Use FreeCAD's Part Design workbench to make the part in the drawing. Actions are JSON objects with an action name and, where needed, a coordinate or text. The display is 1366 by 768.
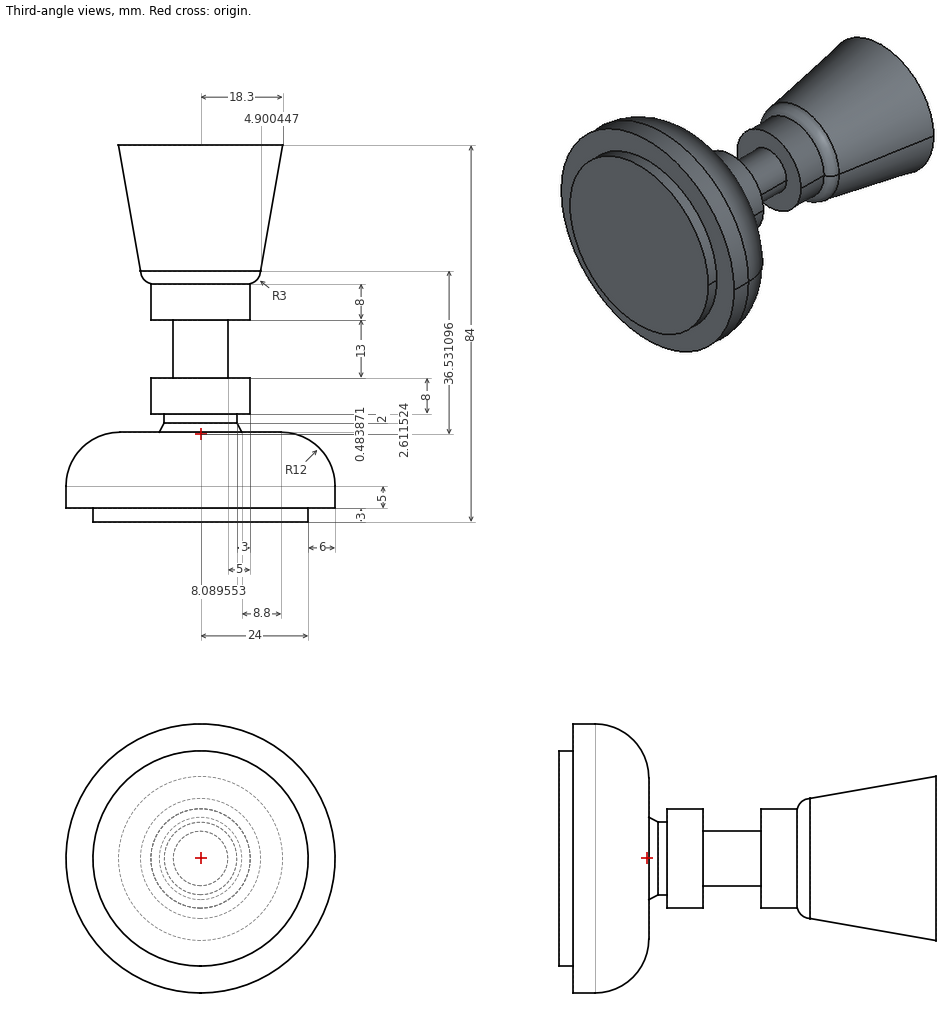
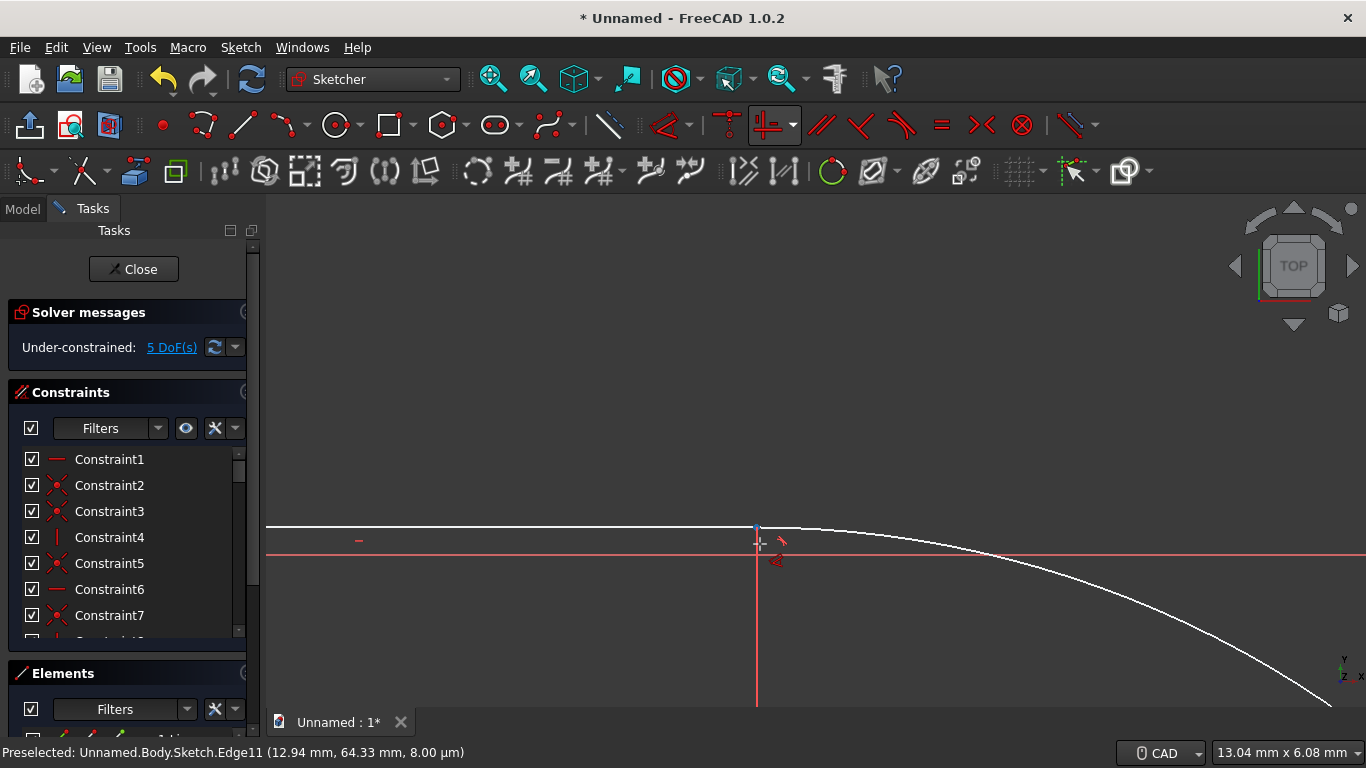
{"action": "left_click", "coordinate": [757, 527]}
{"action": "left_click", "coordinate": [791, 541]}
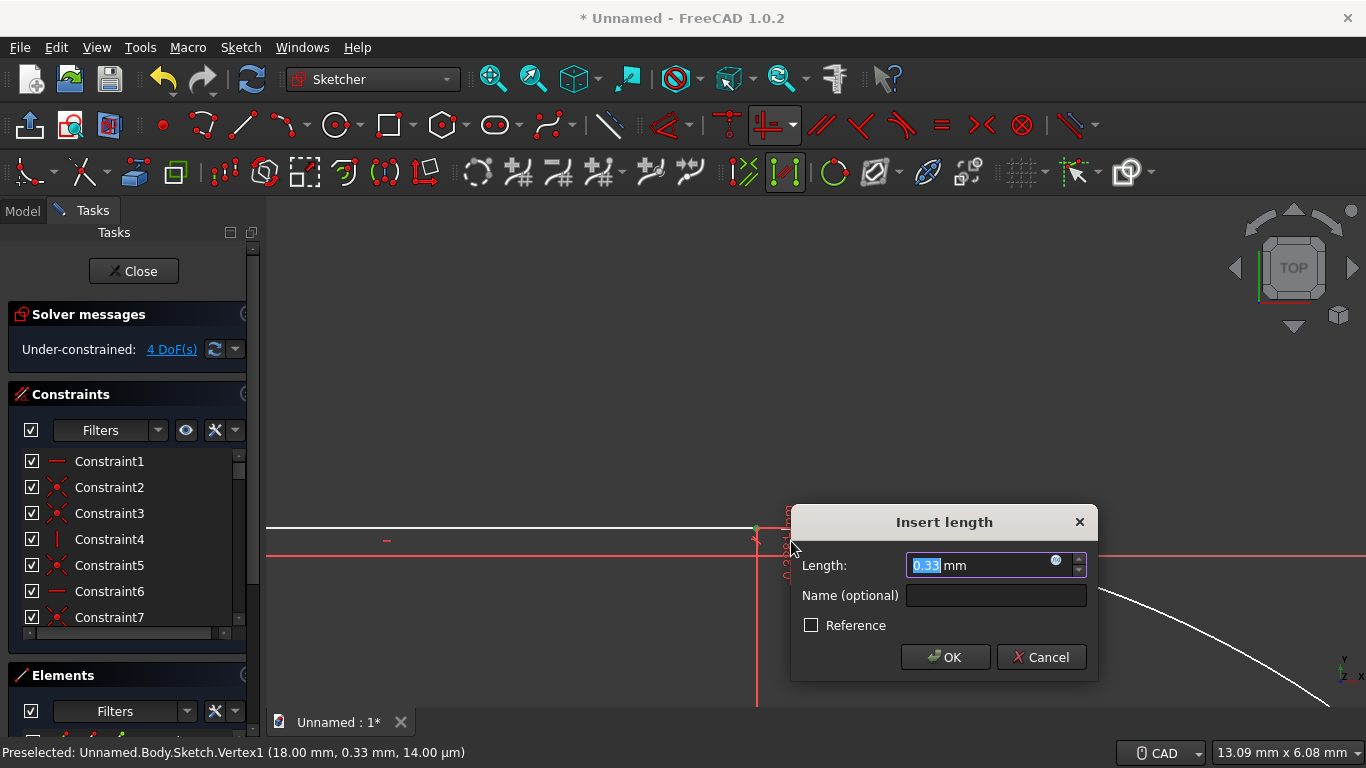
{"action": "type", "text": "0.483871"}
{"action": "key", "text": "Return"}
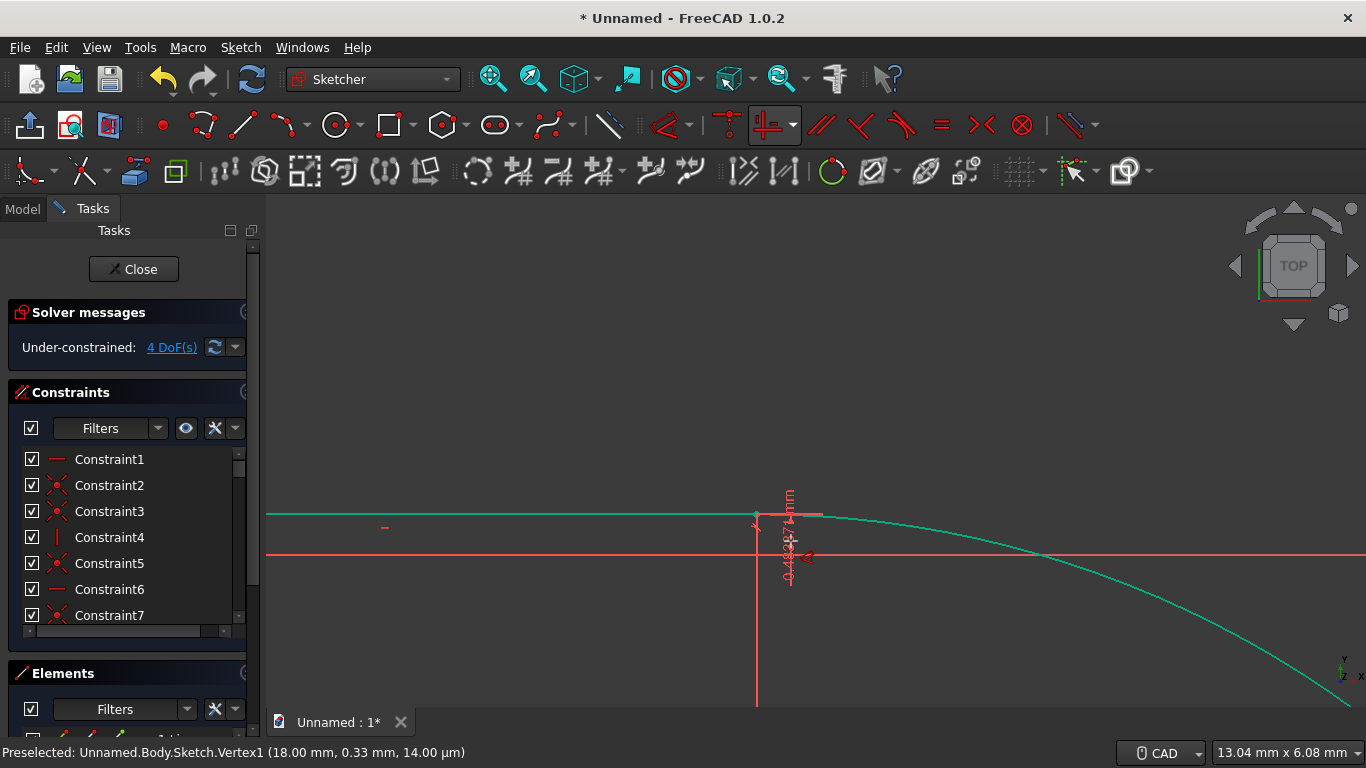
{"action": "scroll", "coordinate": [760, 544], "scroll_direction": "down", "scroll_amount": 15}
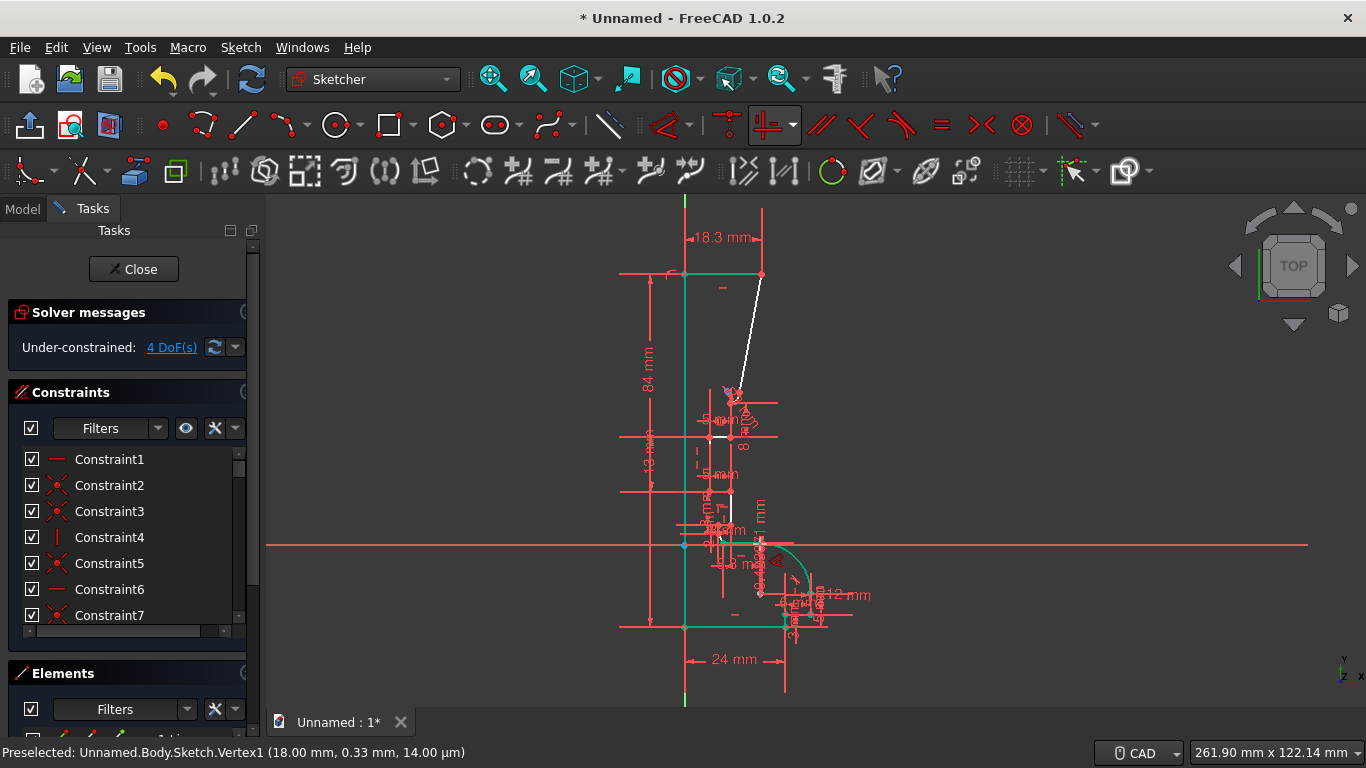
{"action": "scroll", "coordinate": [718, 534], "scroll_direction": "up", "scroll_amount": 2}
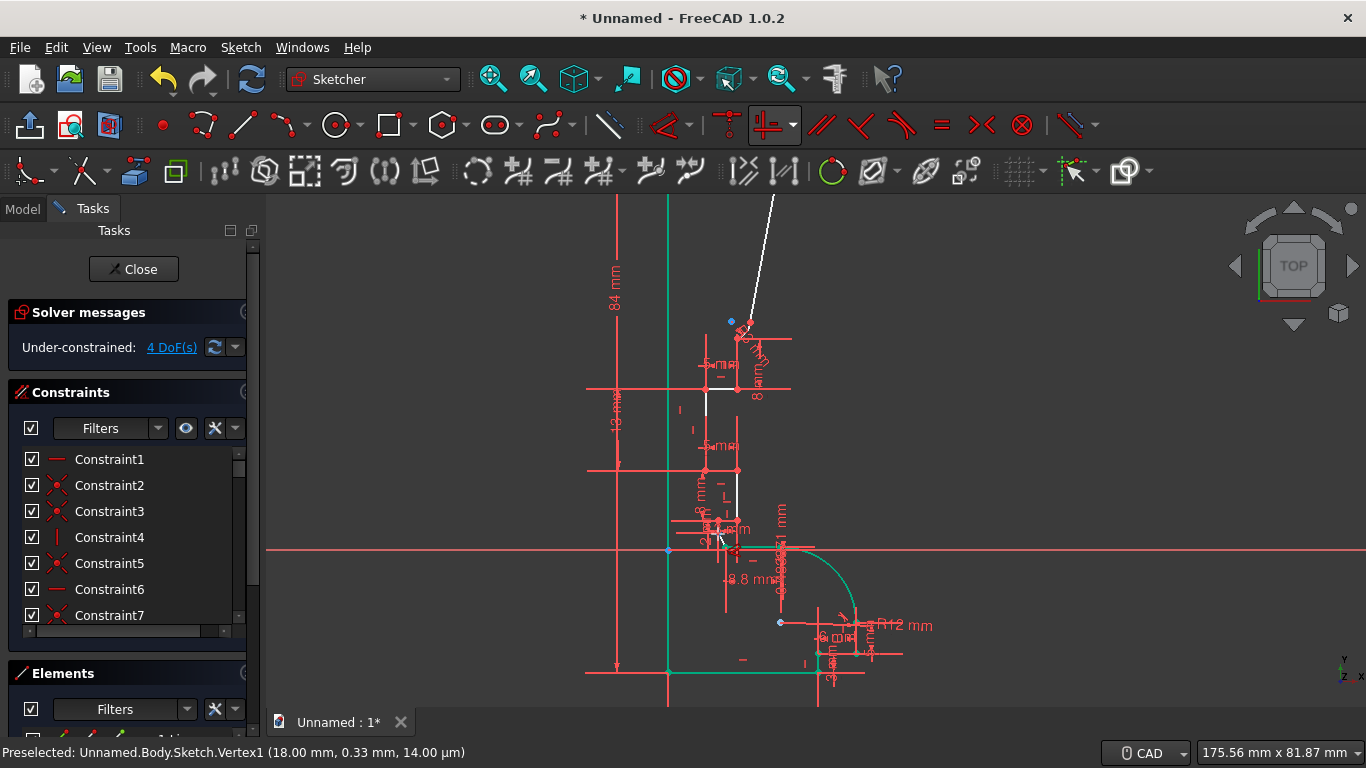
{"action": "left_click", "coordinate": [718, 533]}
{"action": "left_click", "coordinate": [682, 584]}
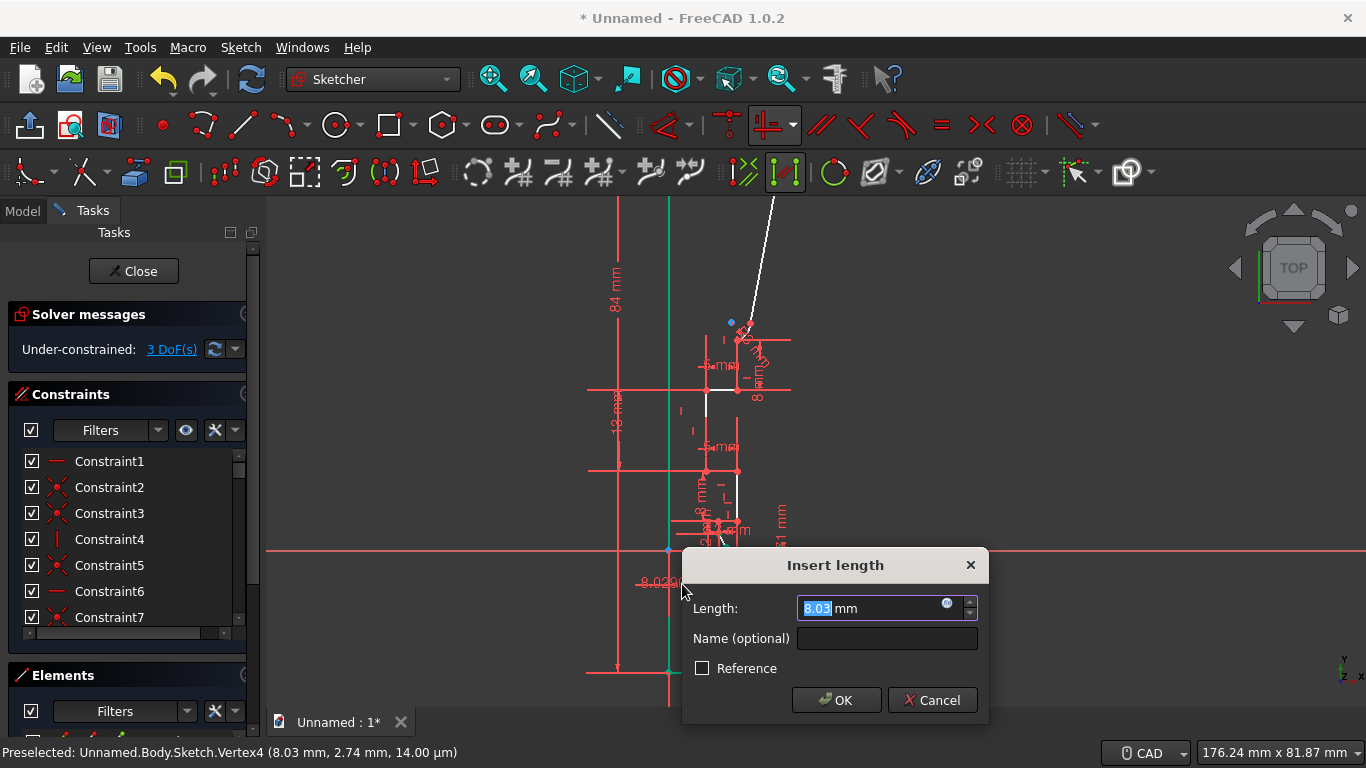
{"action": "type", "text": "8.089553"}
{"action": "key", "text": "Return"}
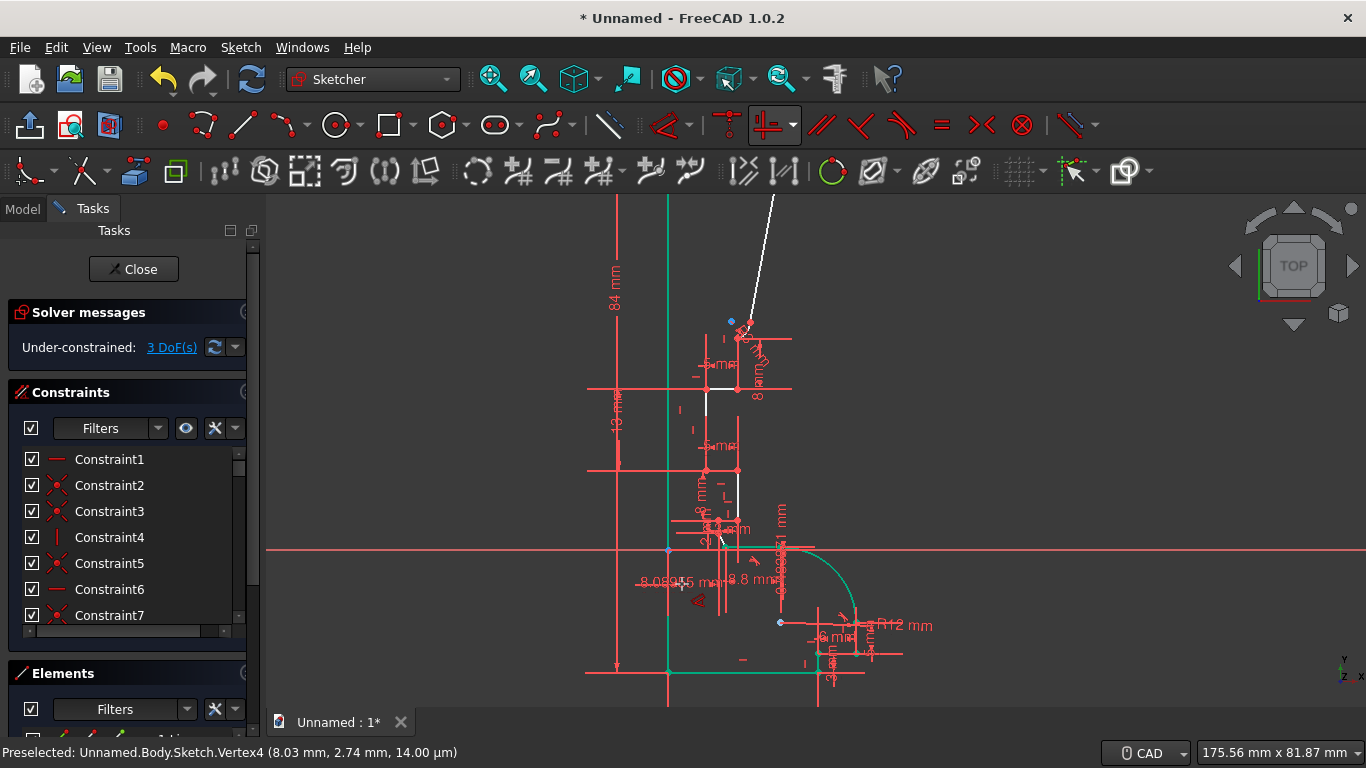
{"action": "scroll", "coordinate": [719, 533], "scroll_direction": "up", "scroll_amount": 5}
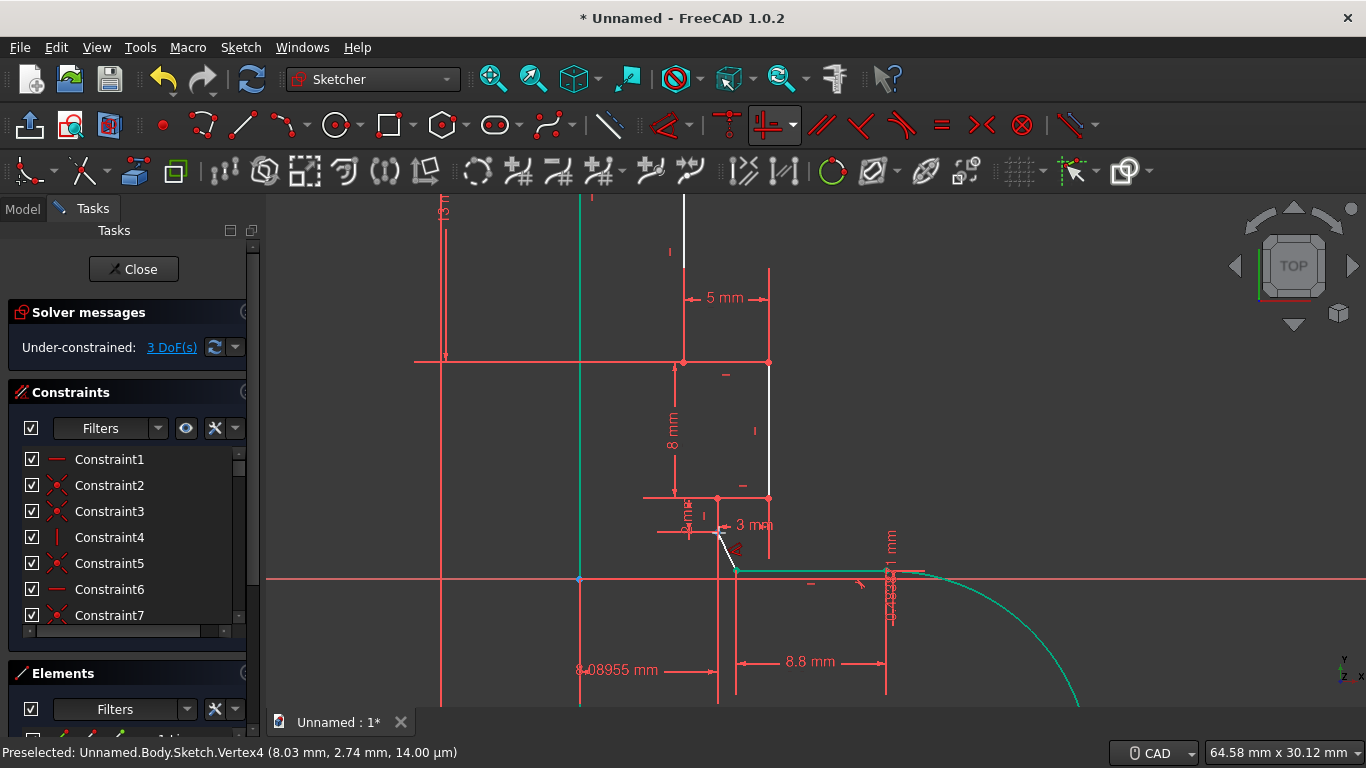
{"action": "left_click", "coordinate": [718, 532]}
{"action": "left_click", "coordinate": [546, 556]}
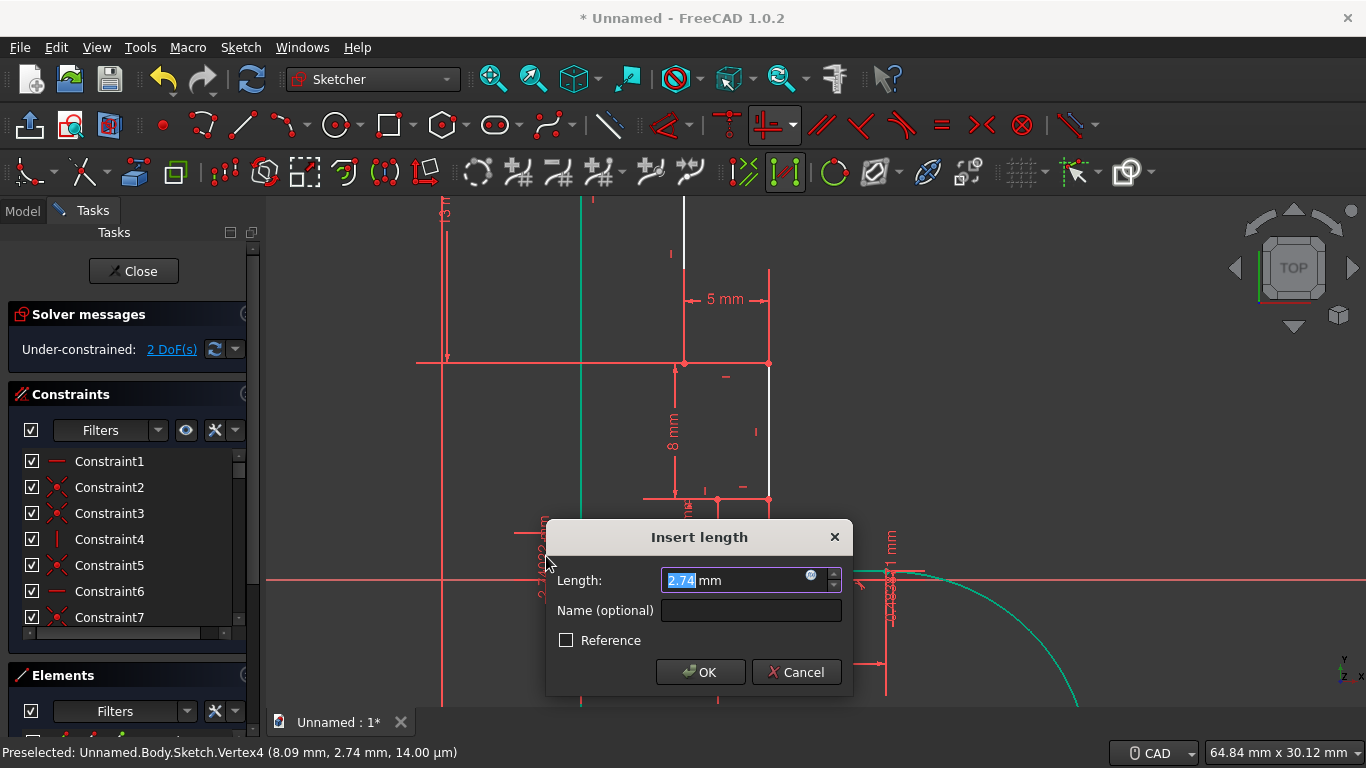
{"action": "type", "text": "2.611524"}
{"action": "key", "text": "Return"}